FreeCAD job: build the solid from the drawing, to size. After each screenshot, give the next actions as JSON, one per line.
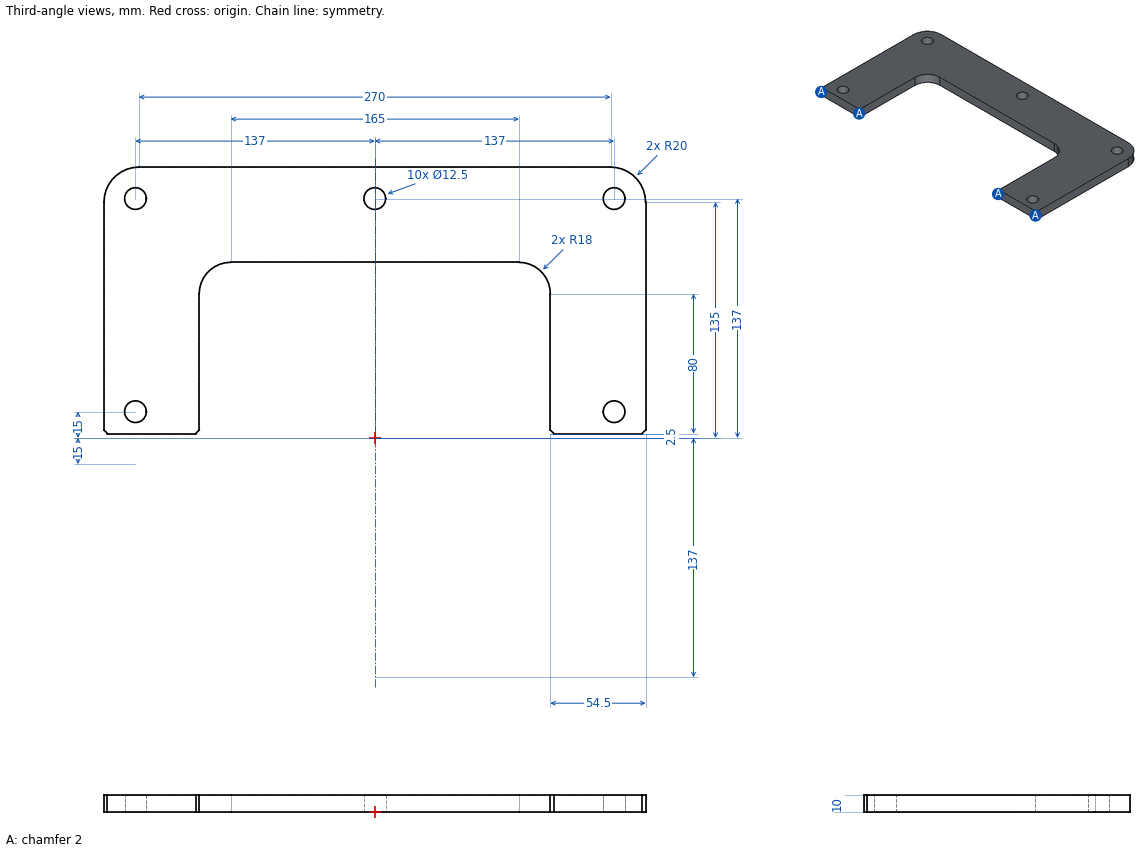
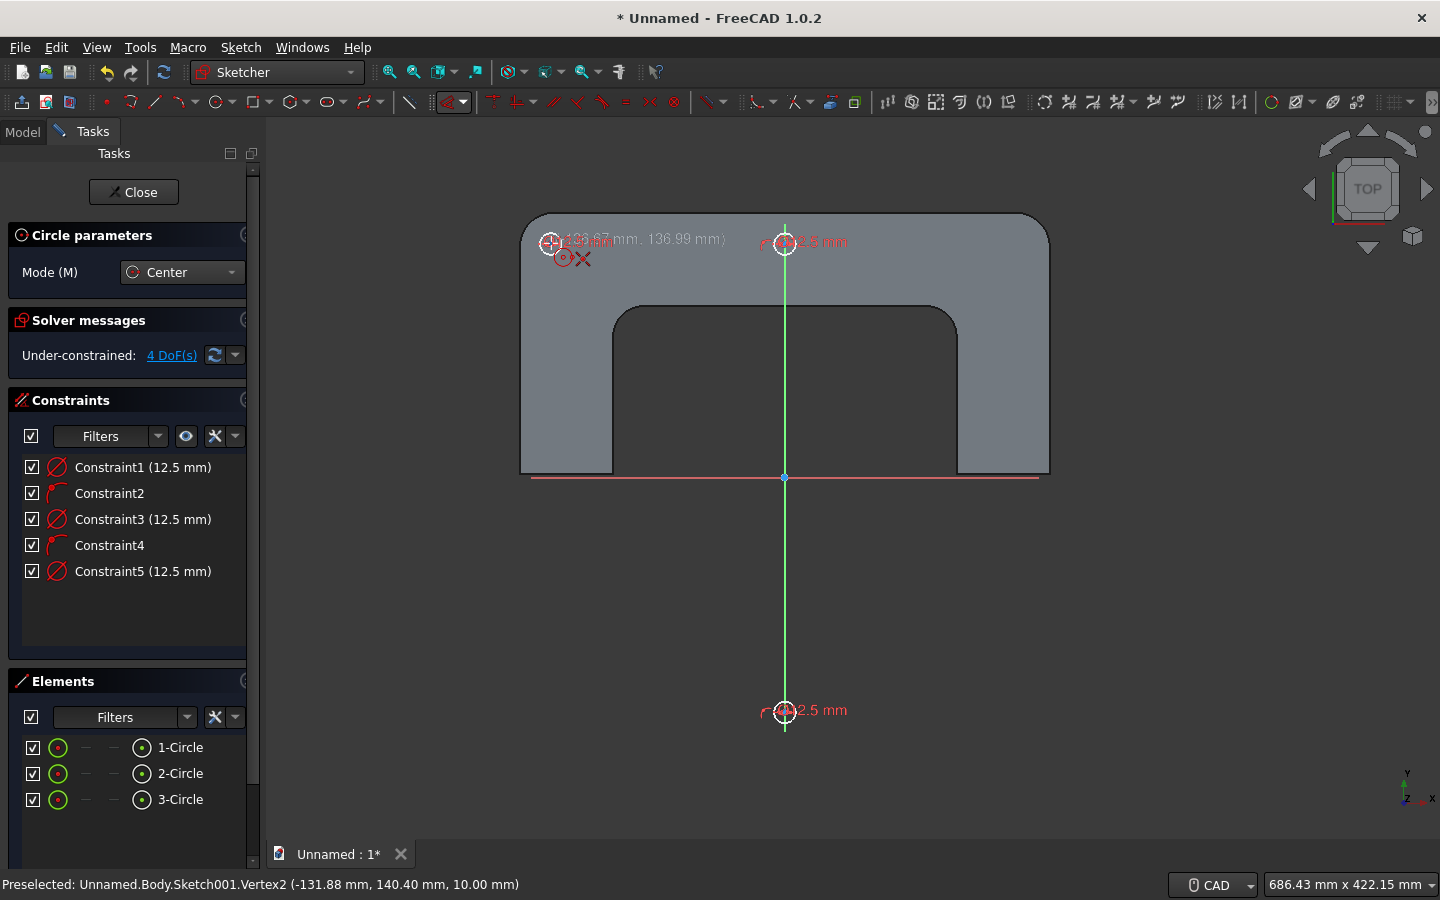
{"action": "scroll", "coordinate": [1019, 244], "scroll_direction": "up", "scroll_amount": 4}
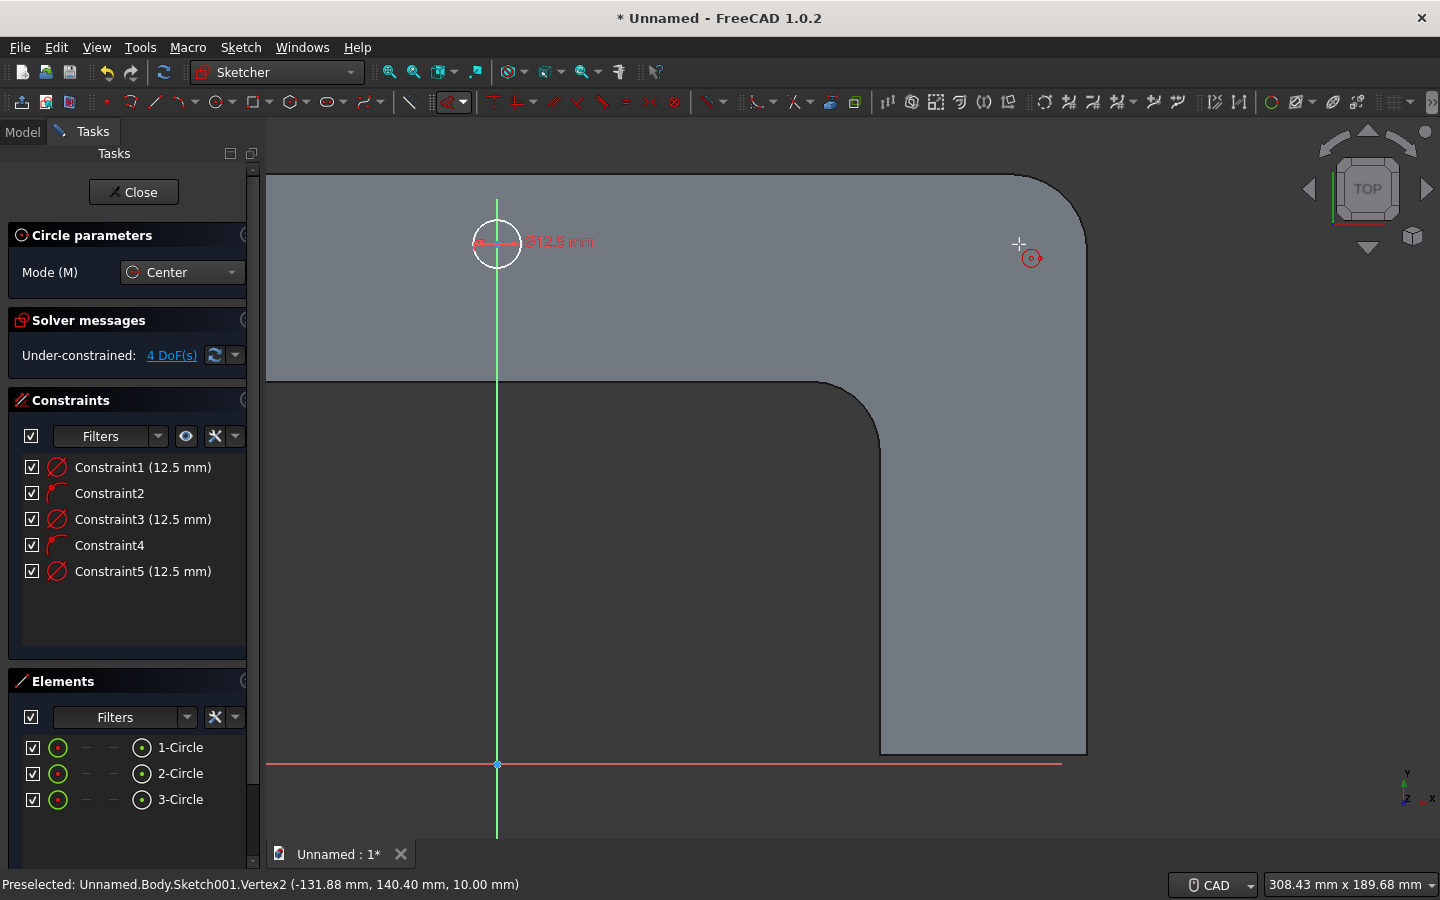
{"action": "left_click", "coordinate": [1019, 243]}
{"action": "mouse_move", "coordinate": [1035, 226]}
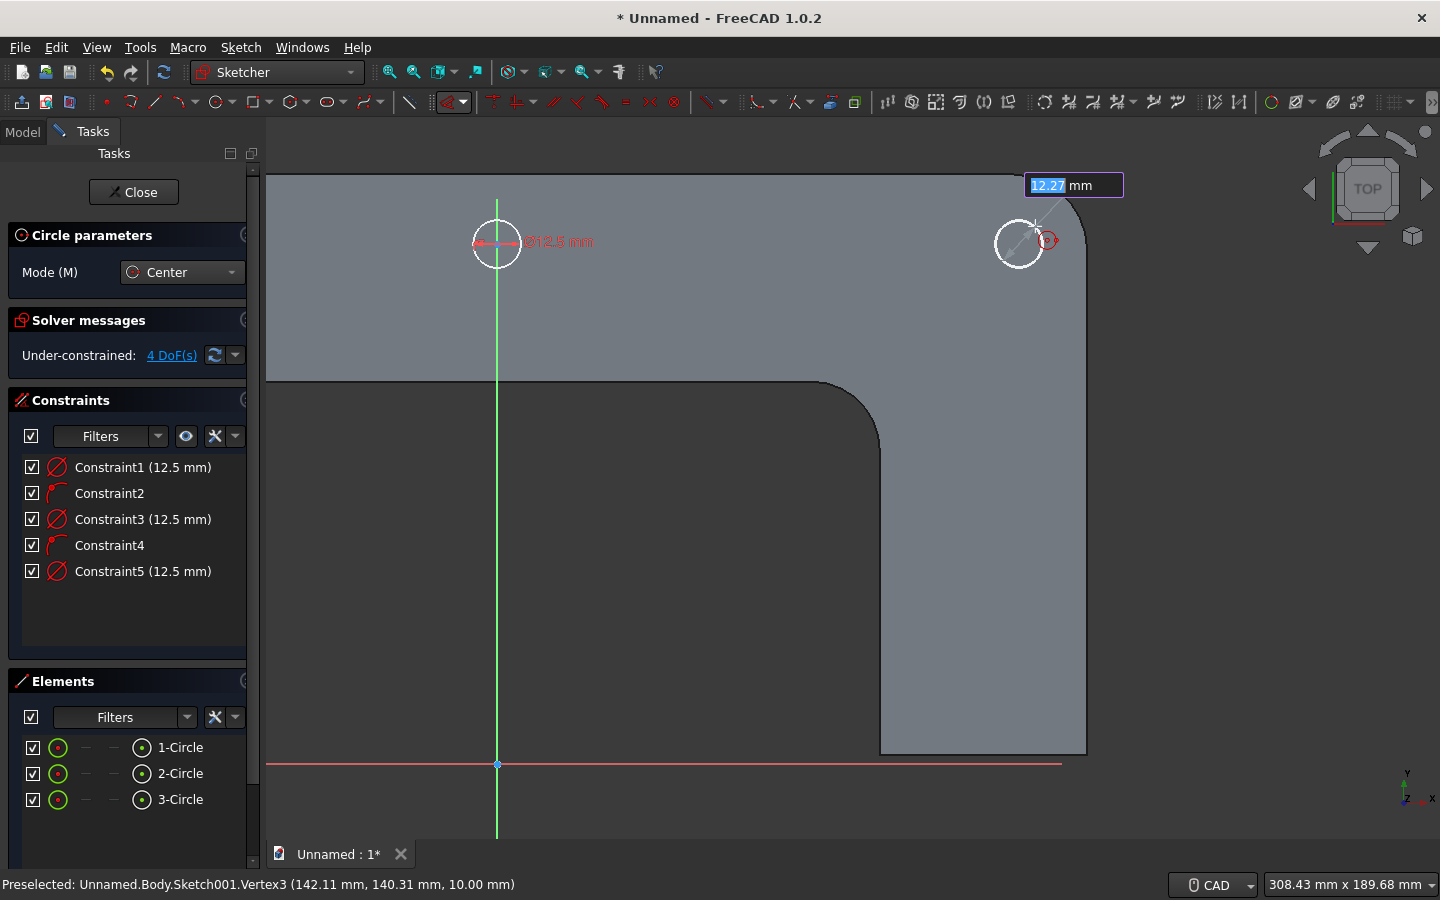
{"action": "type", "text": "12.5"}
{"action": "key", "text": "Return"}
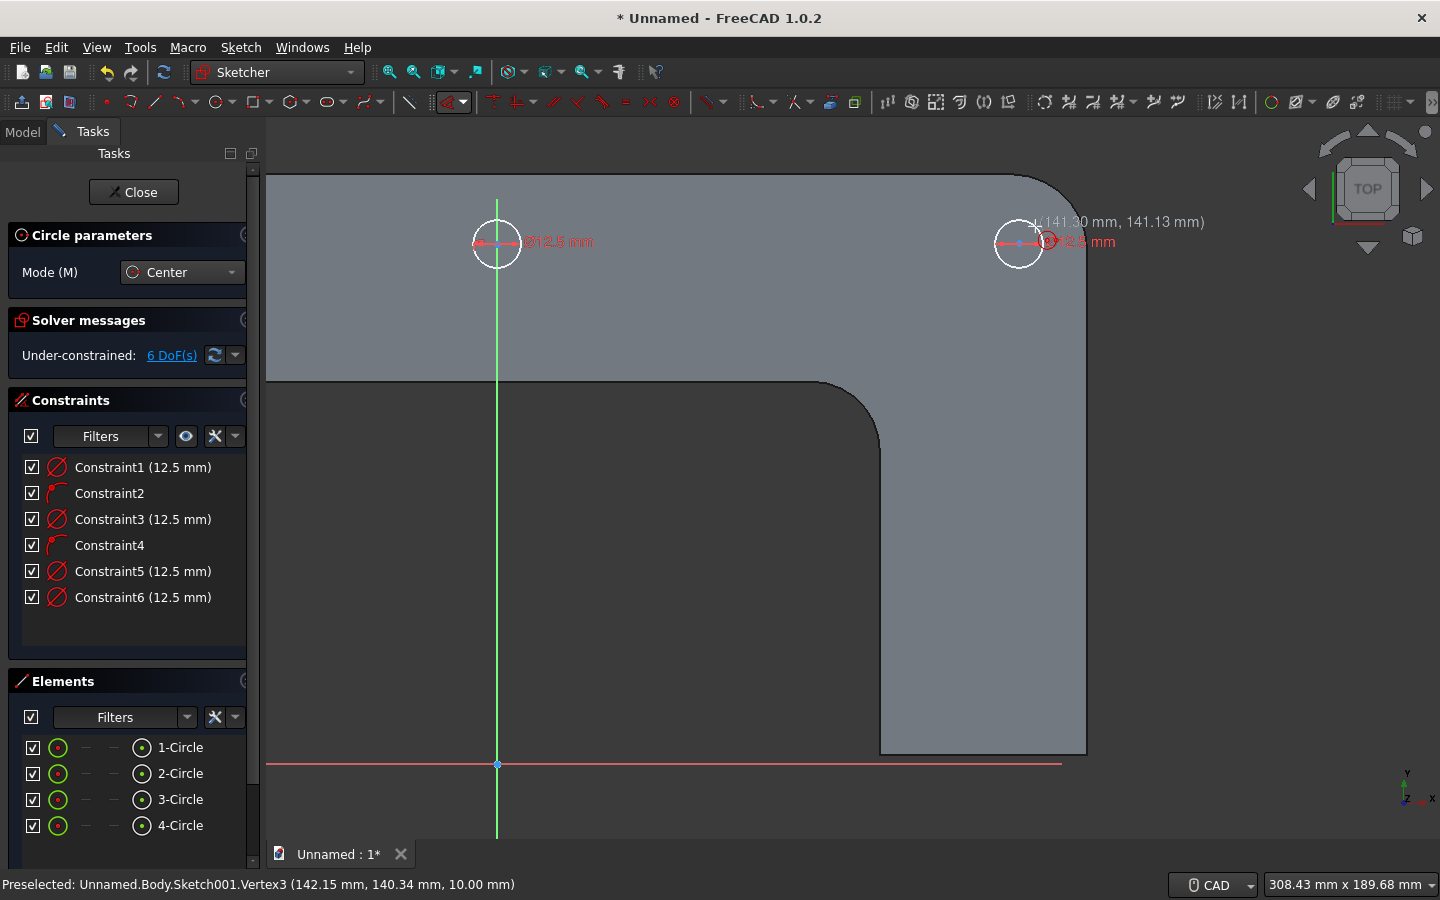
{"action": "scroll", "coordinate": [1019, 244], "scroll_direction": "down", "scroll_amount": 4}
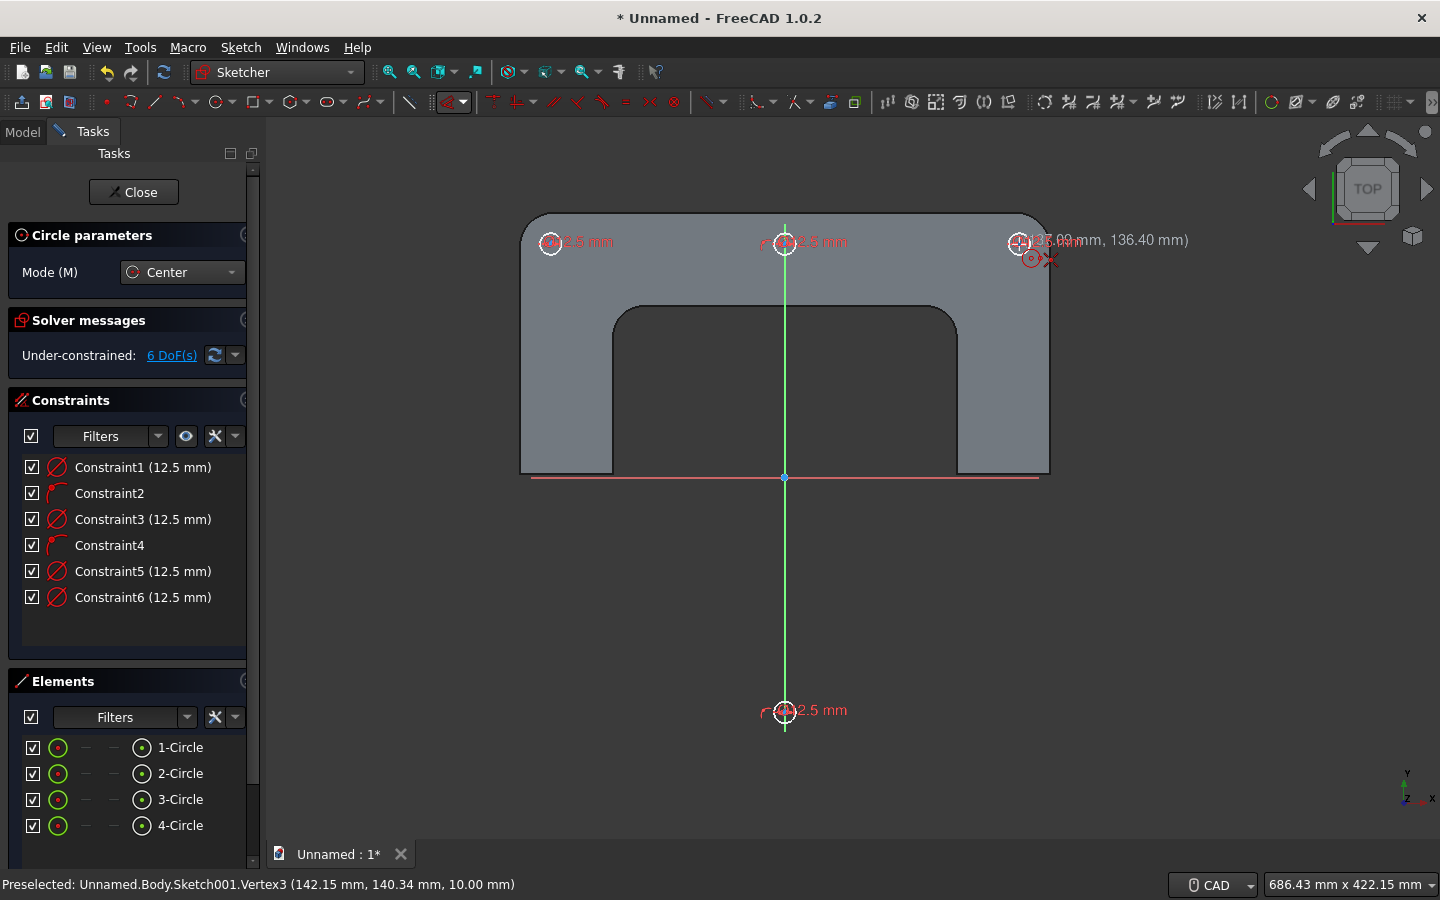
{"action": "scroll", "coordinate": [551, 712], "scroll_direction": "up", "scroll_amount": 4}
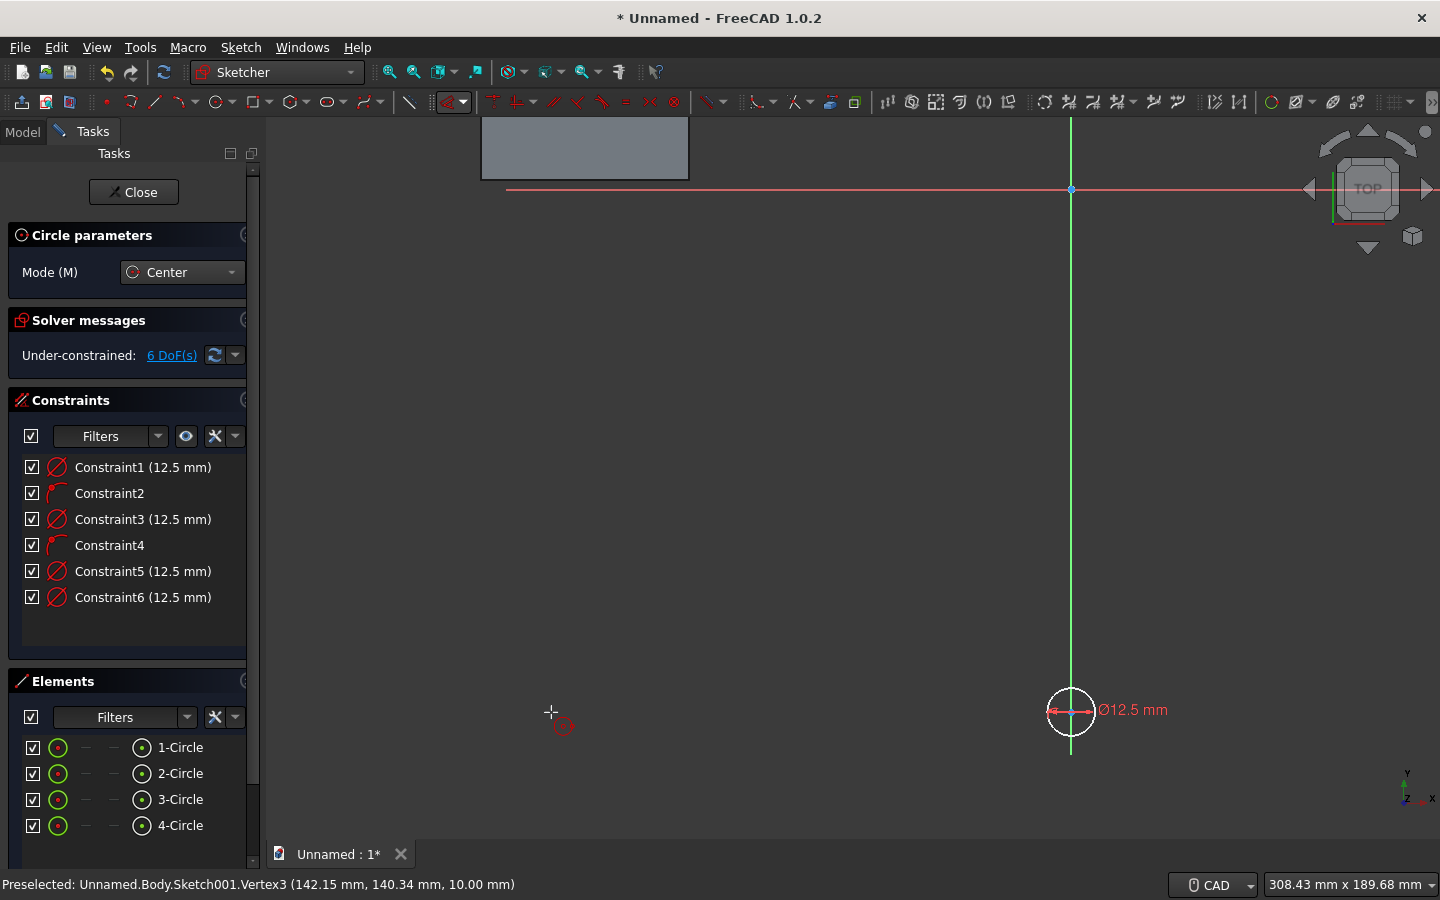
{"action": "left_click", "coordinate": [550, 711]}
{"action": "mouse_move", "coordinate": [567, 694]}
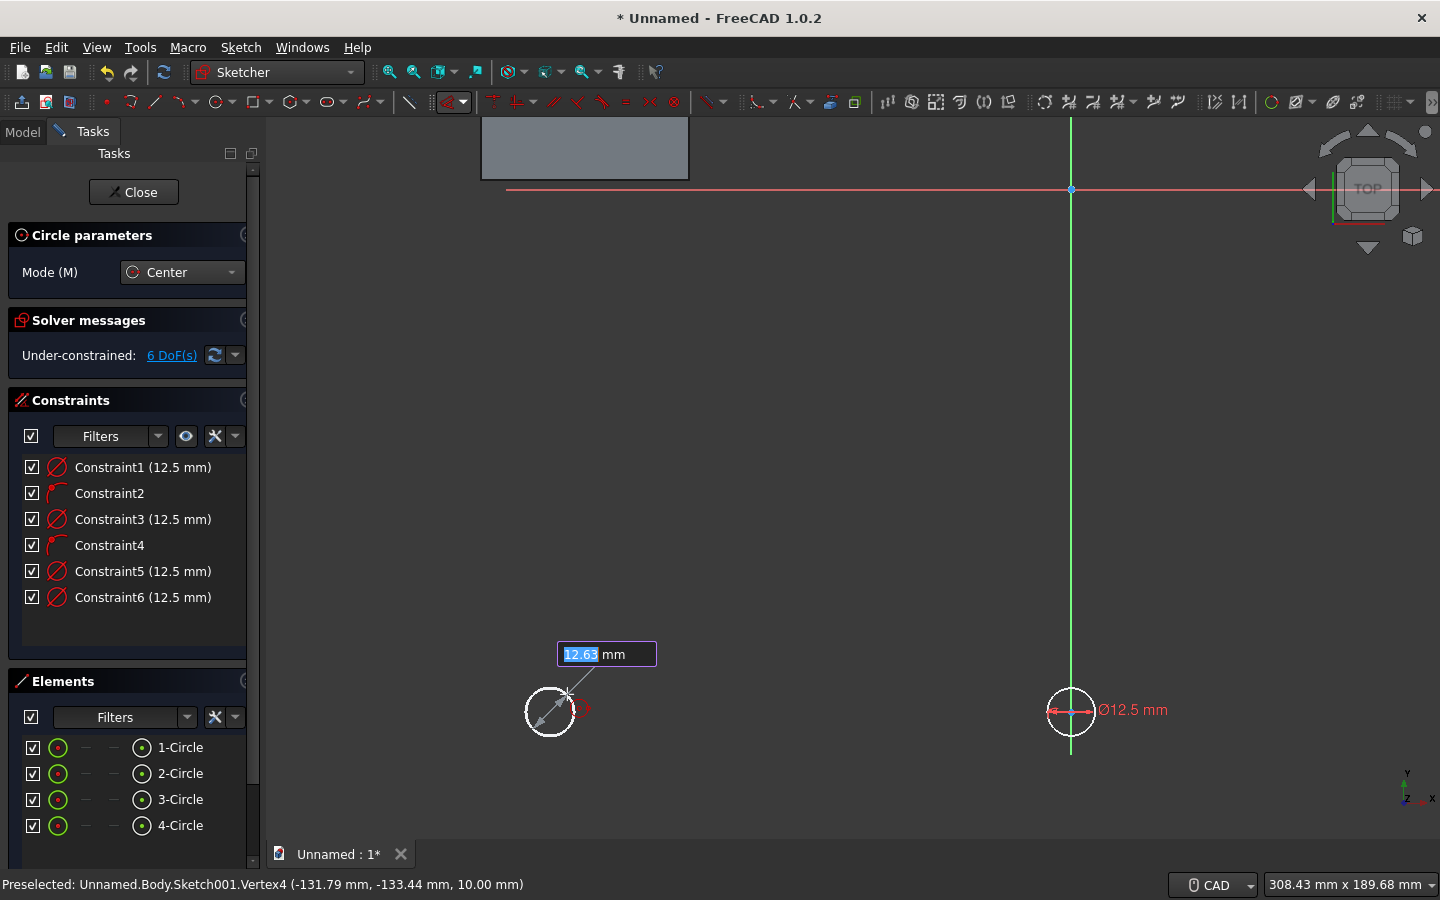
{"action": "type", "text": "12.5"}
{"action": "key", "text": "Return"}